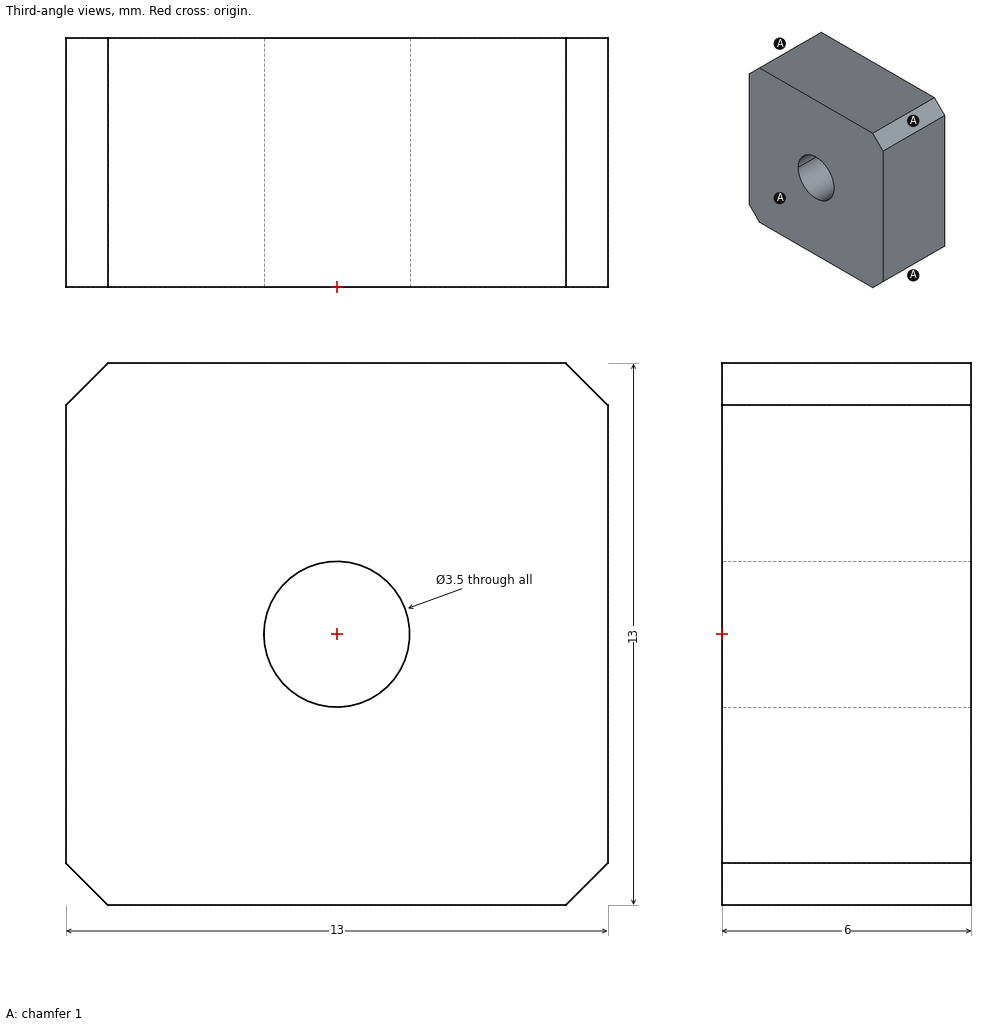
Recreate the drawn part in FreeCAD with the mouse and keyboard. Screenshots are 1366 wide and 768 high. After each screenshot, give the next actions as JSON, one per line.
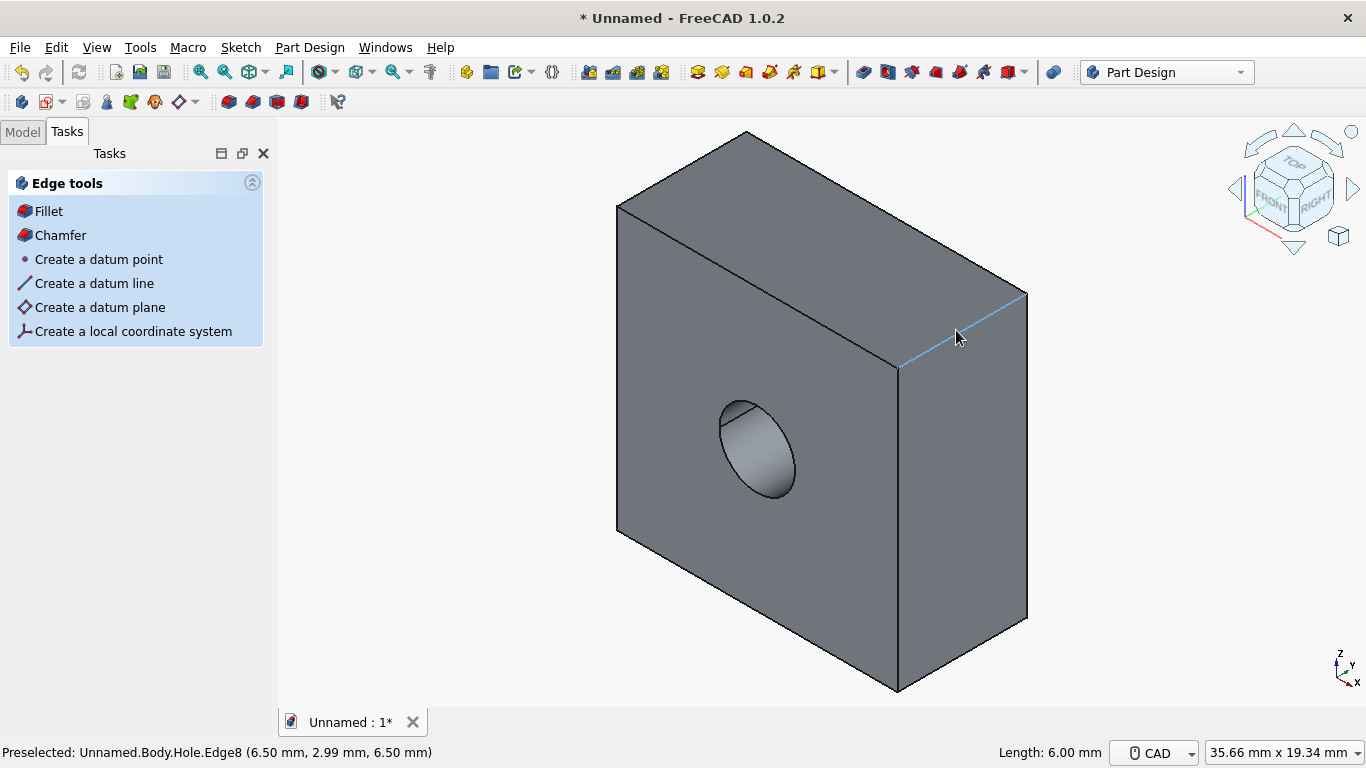
{"action": "key", "text": "2"}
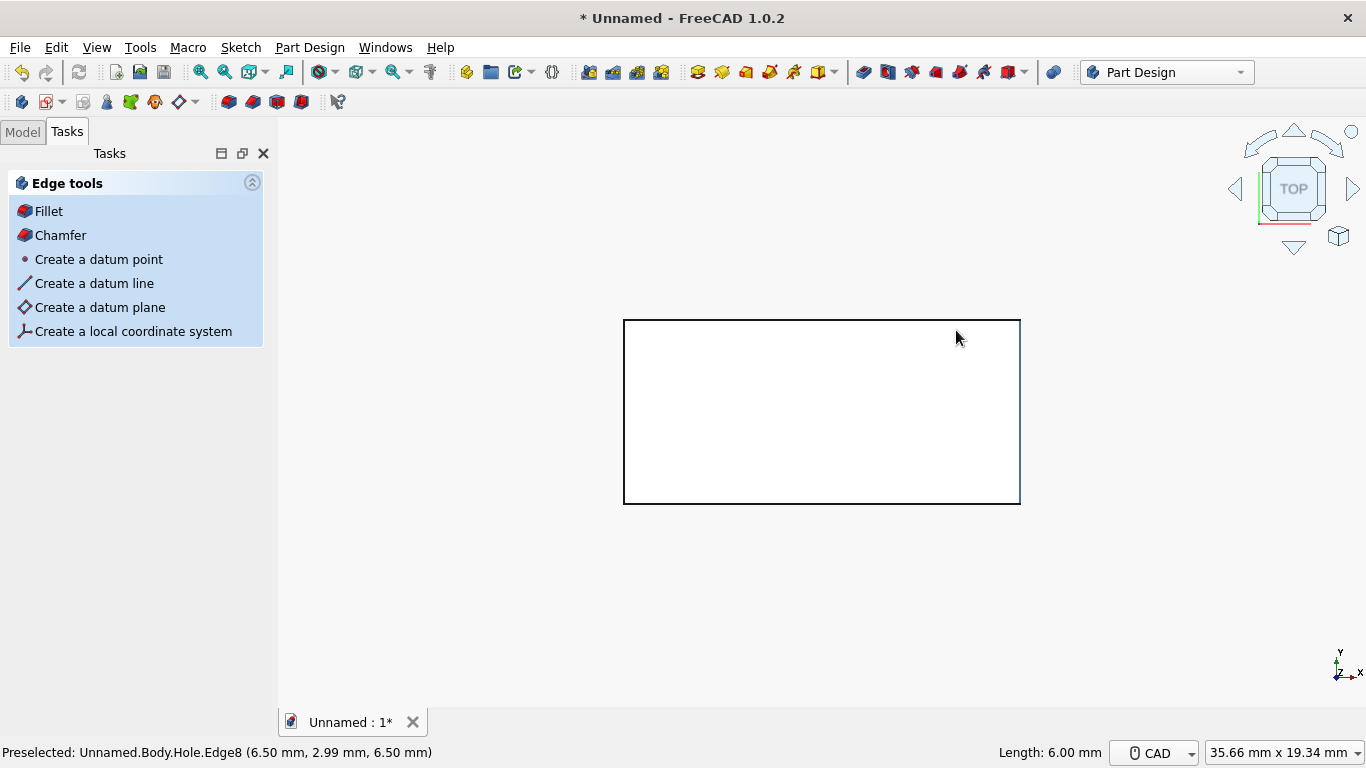
{"action": "left_click", "coordinate": [202, 72]}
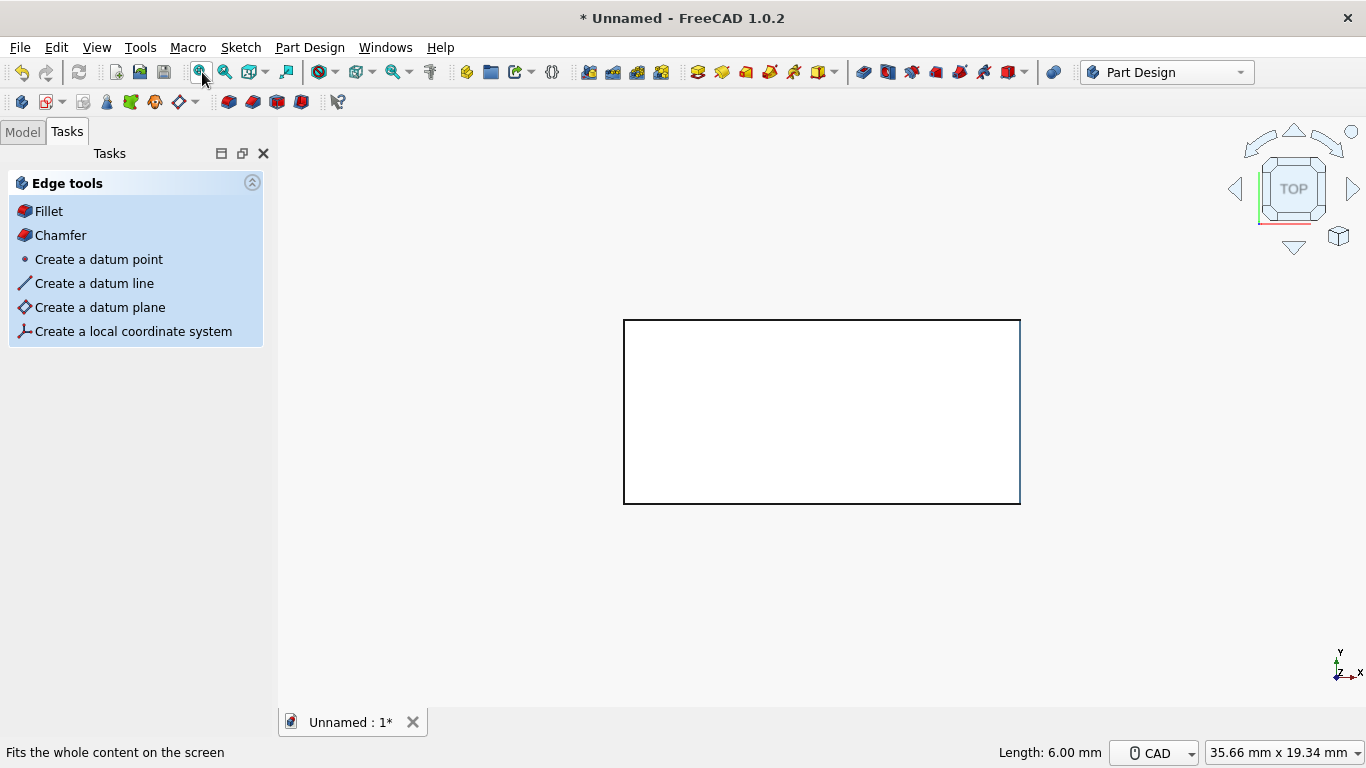
{"action": "left_click", "coordinate": [624, 411], "text": "ctrl"}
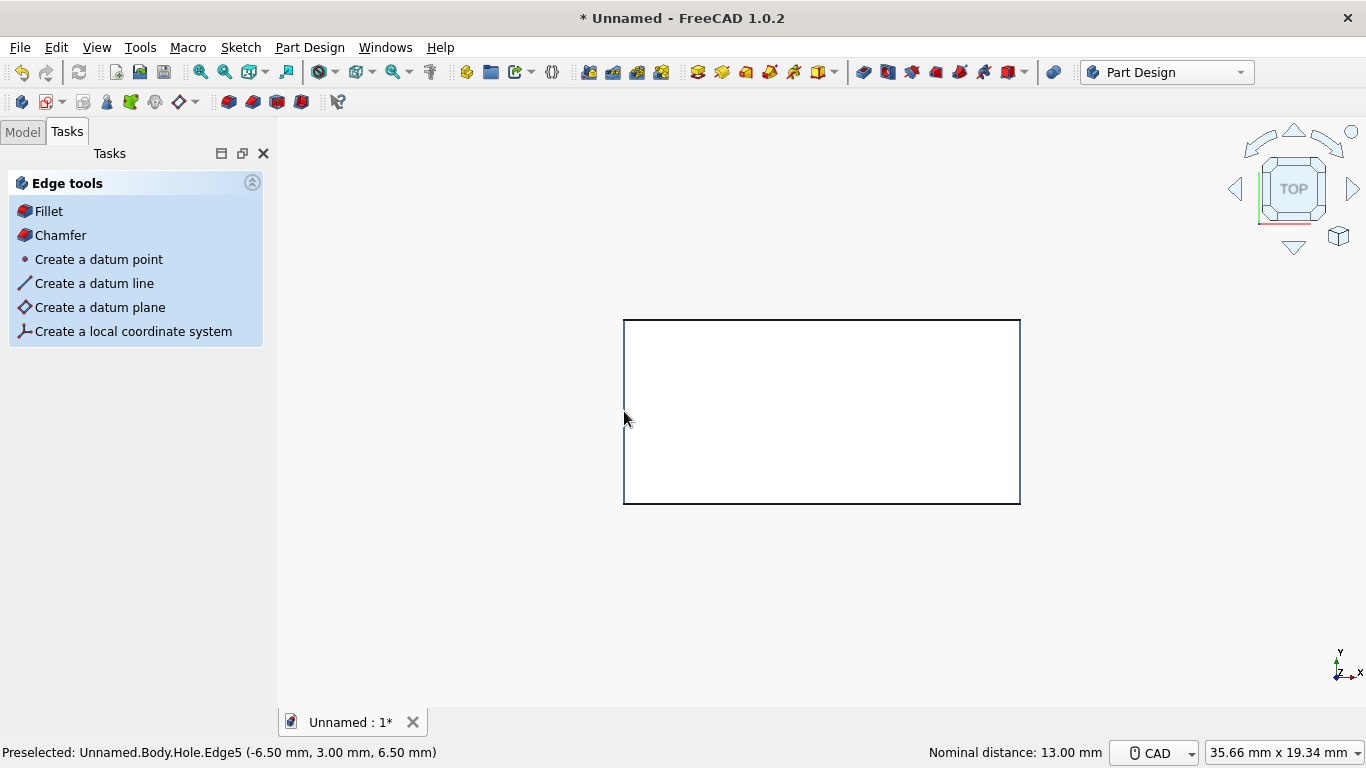
{"action": "key", "text": "1"}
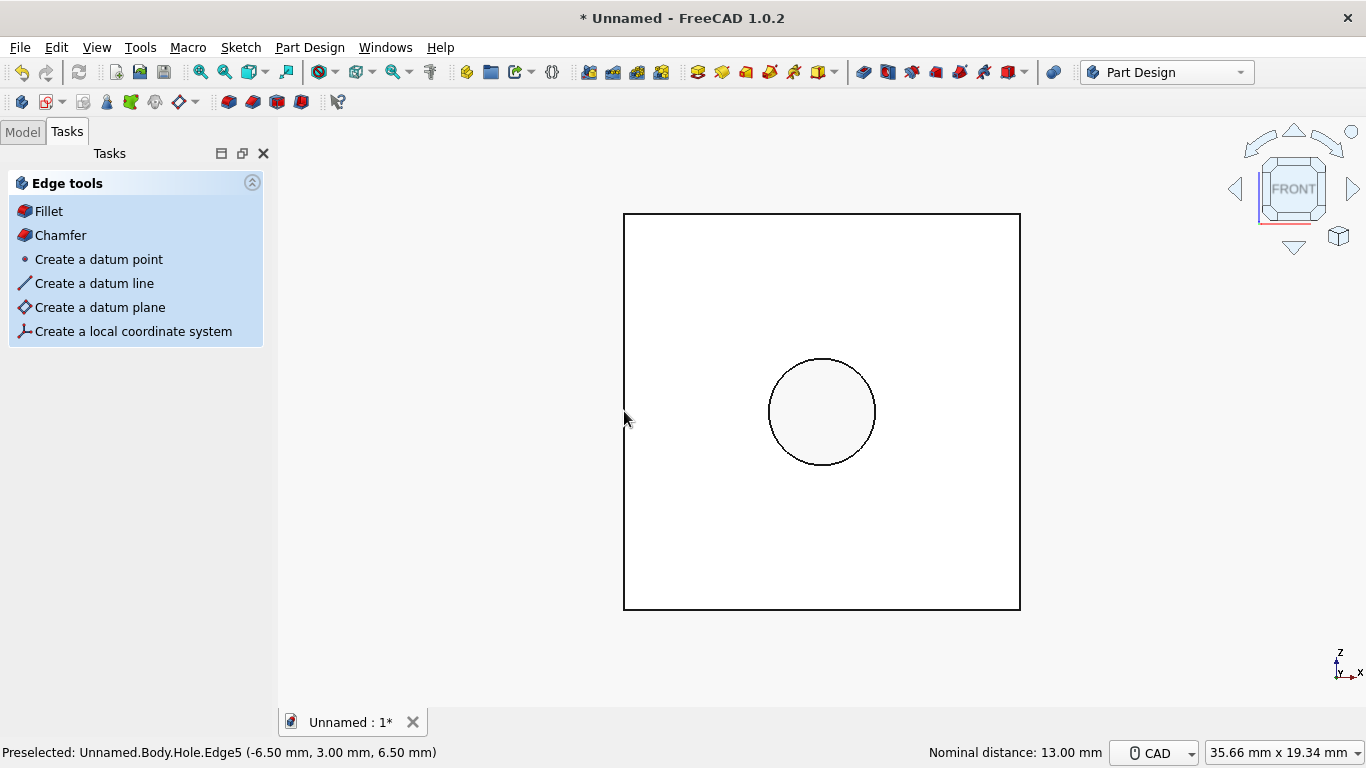
{"action": "key", "text": "3"}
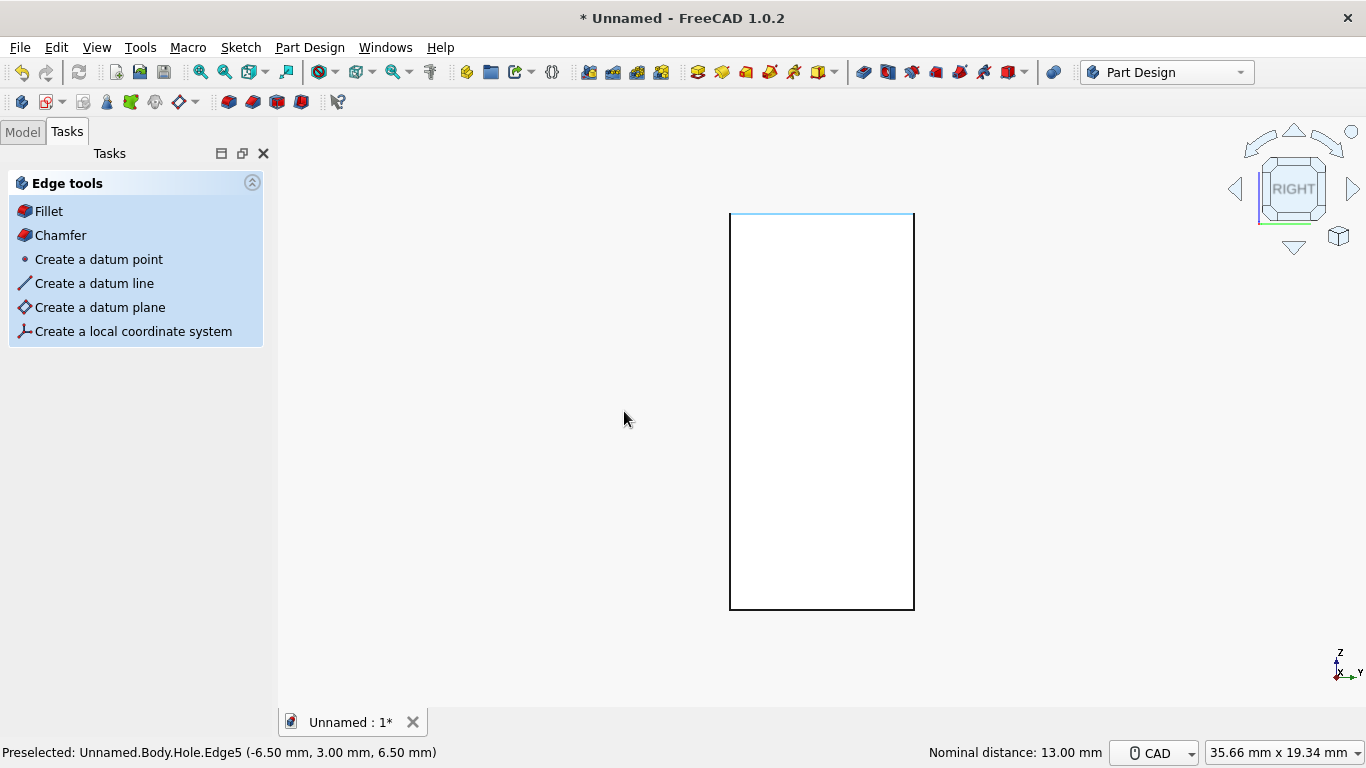
{"action": "left_click", "coordinate": [822, 609], "text": "ctrl"}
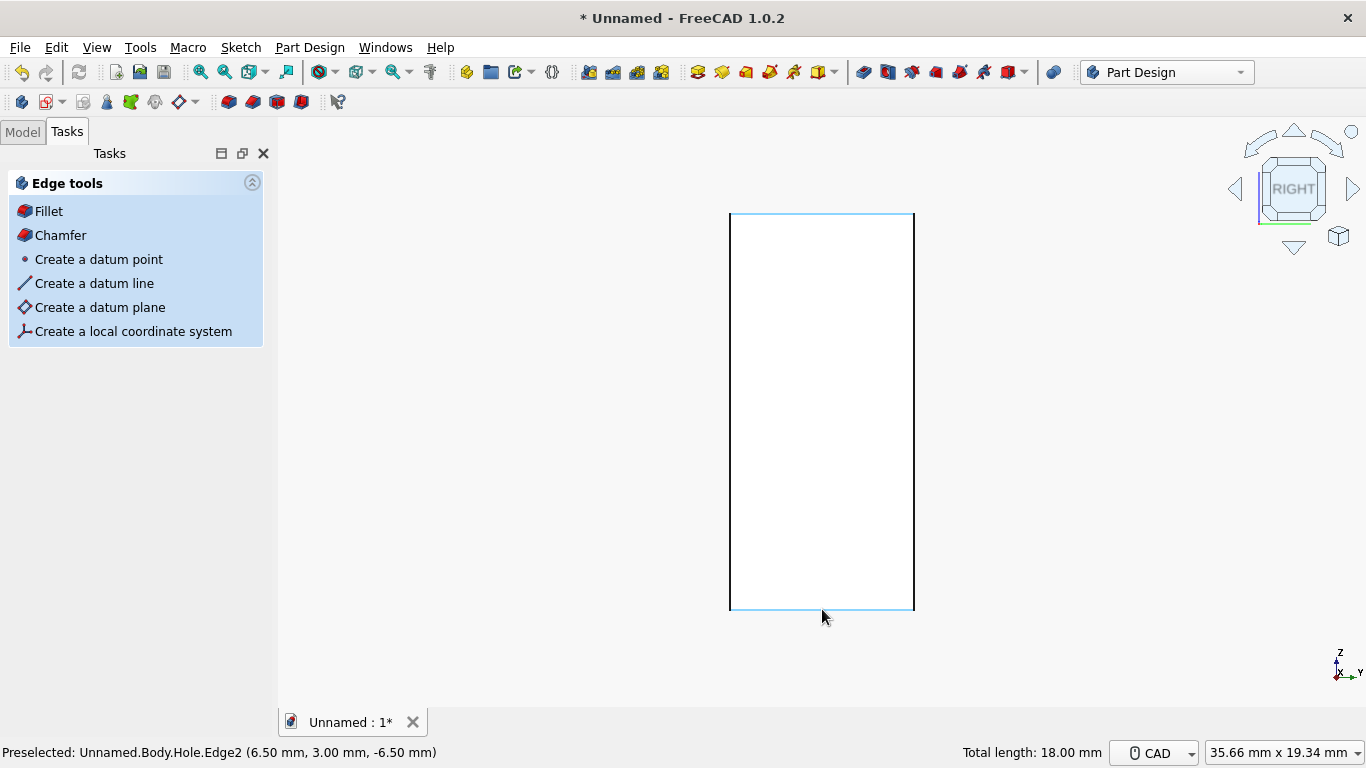
{"action": "key", "text": "5"}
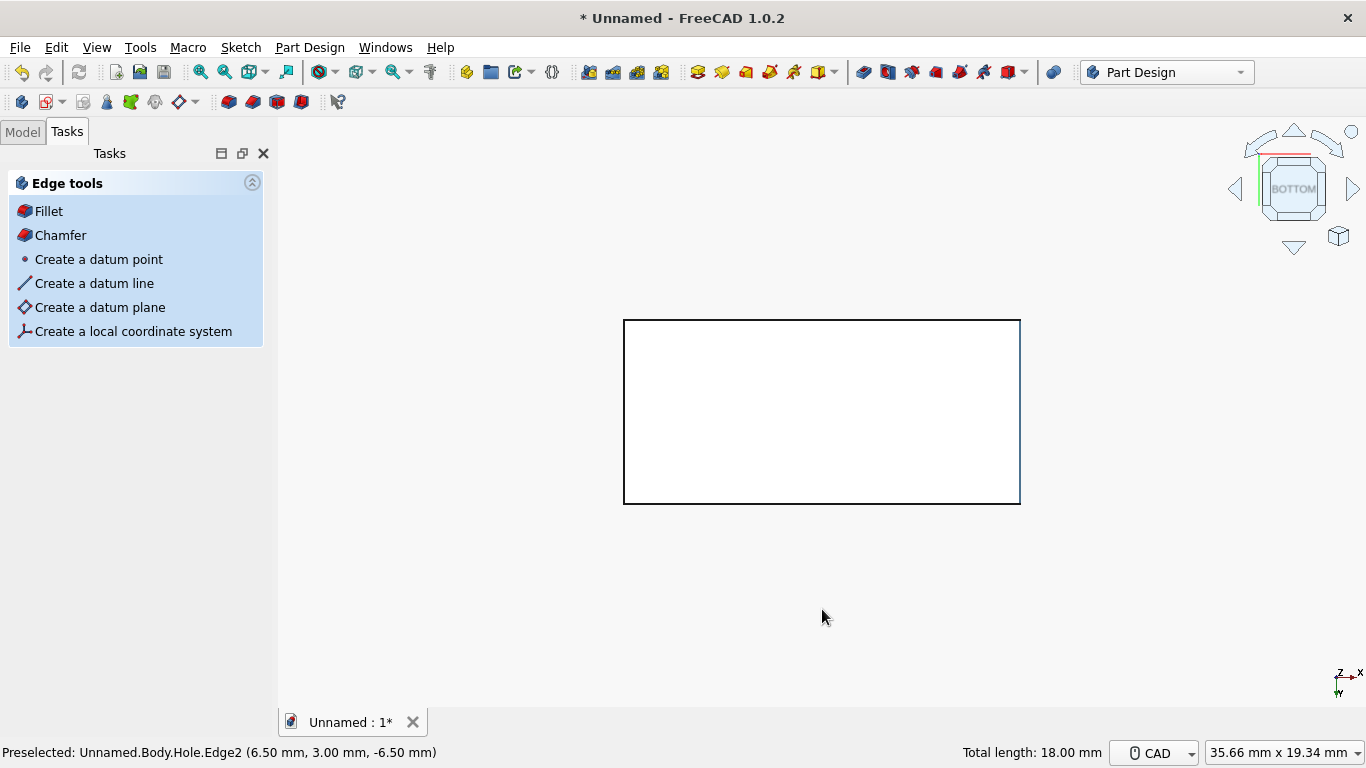
{"action": "key", "text": "v f"}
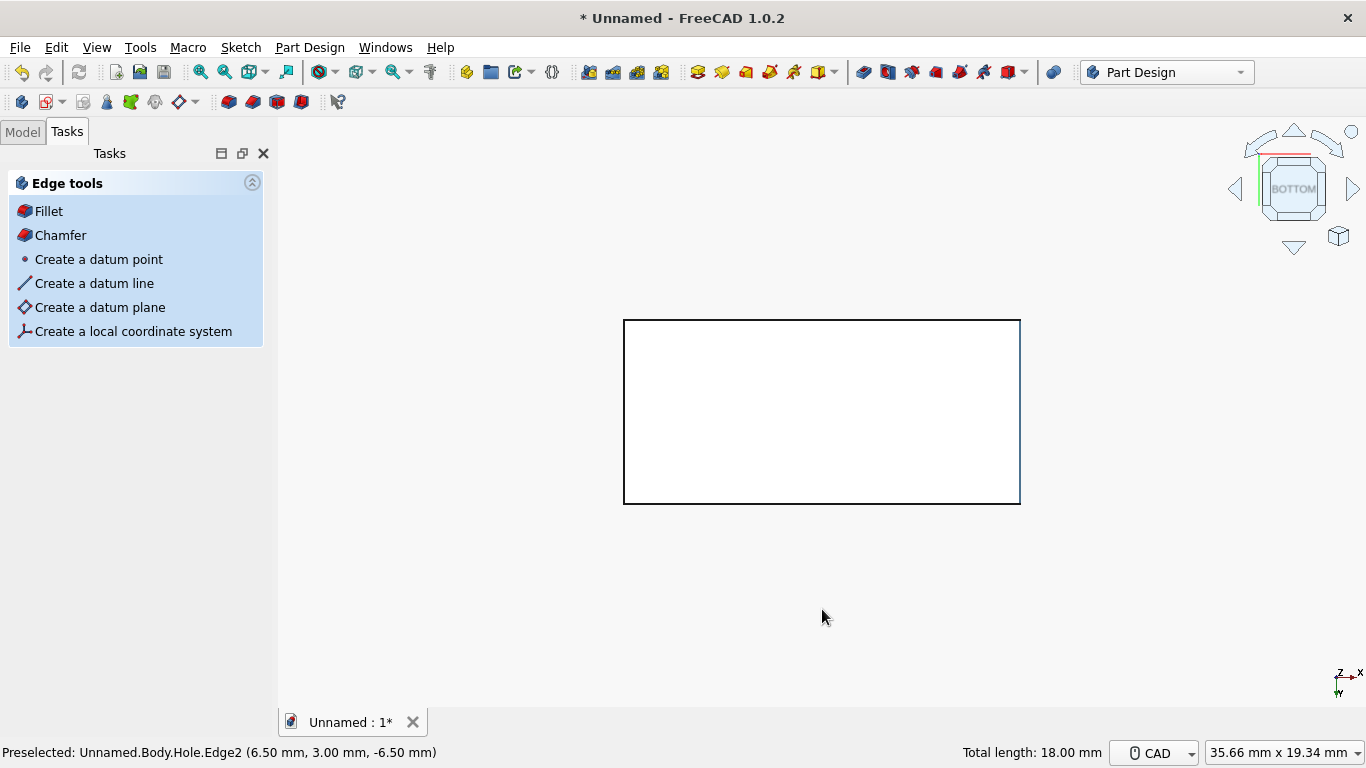
{"action": "left_click", "coordinate": [624, 411], "text": "ctrl"}